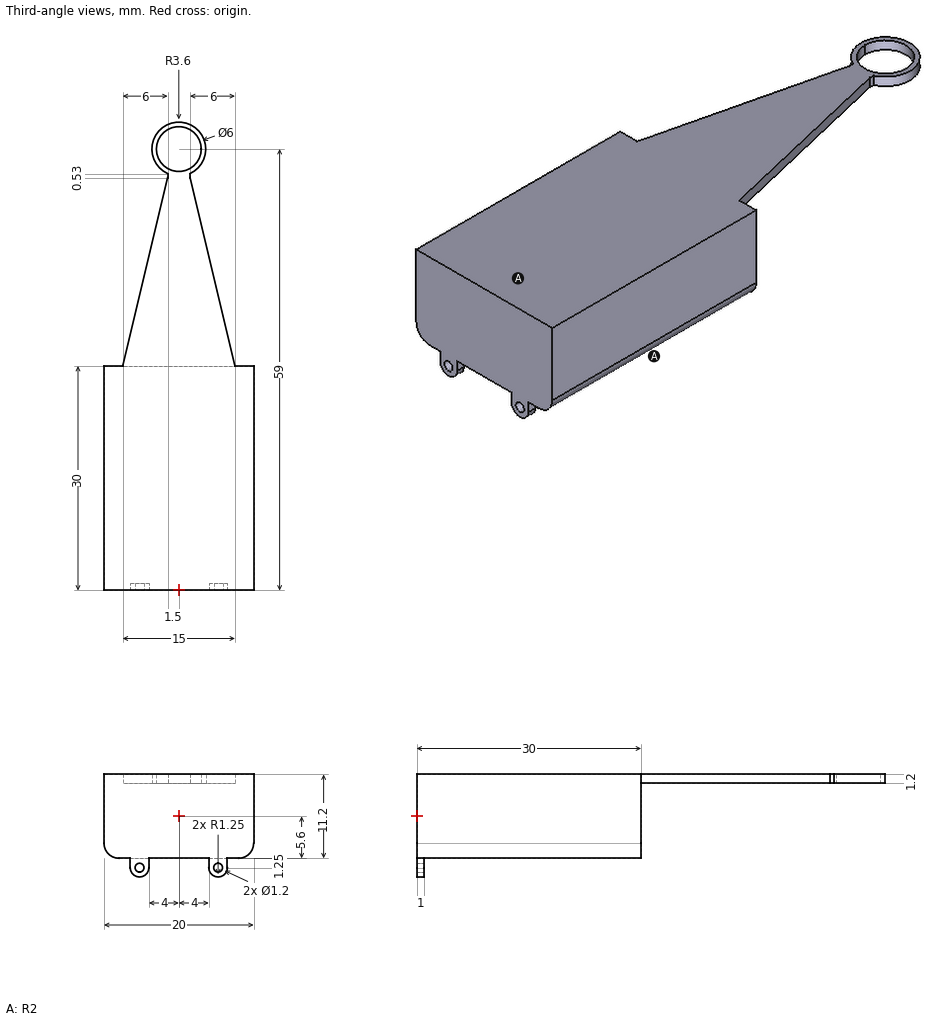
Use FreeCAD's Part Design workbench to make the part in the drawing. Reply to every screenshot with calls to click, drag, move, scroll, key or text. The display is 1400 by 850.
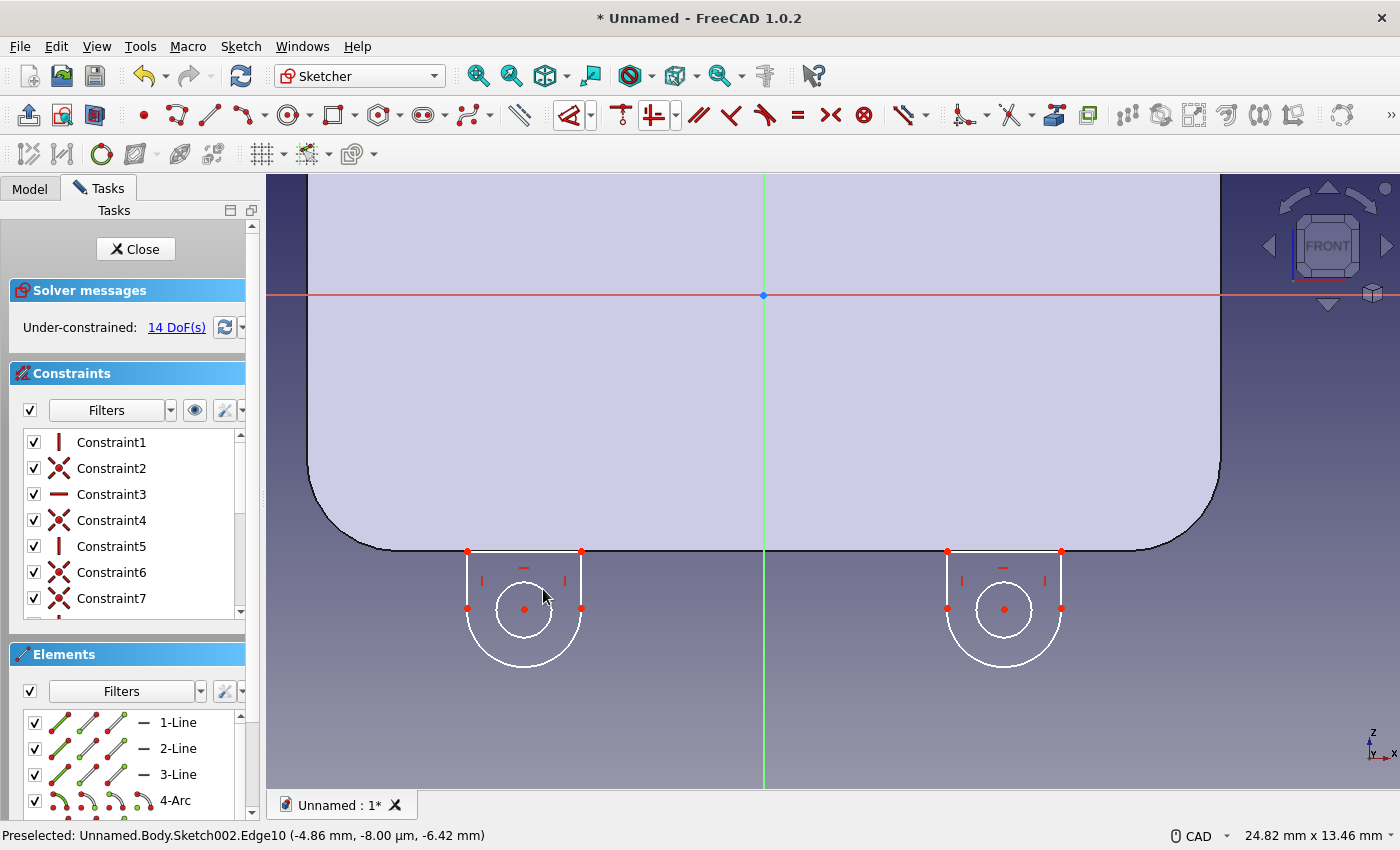
click(1061, 592)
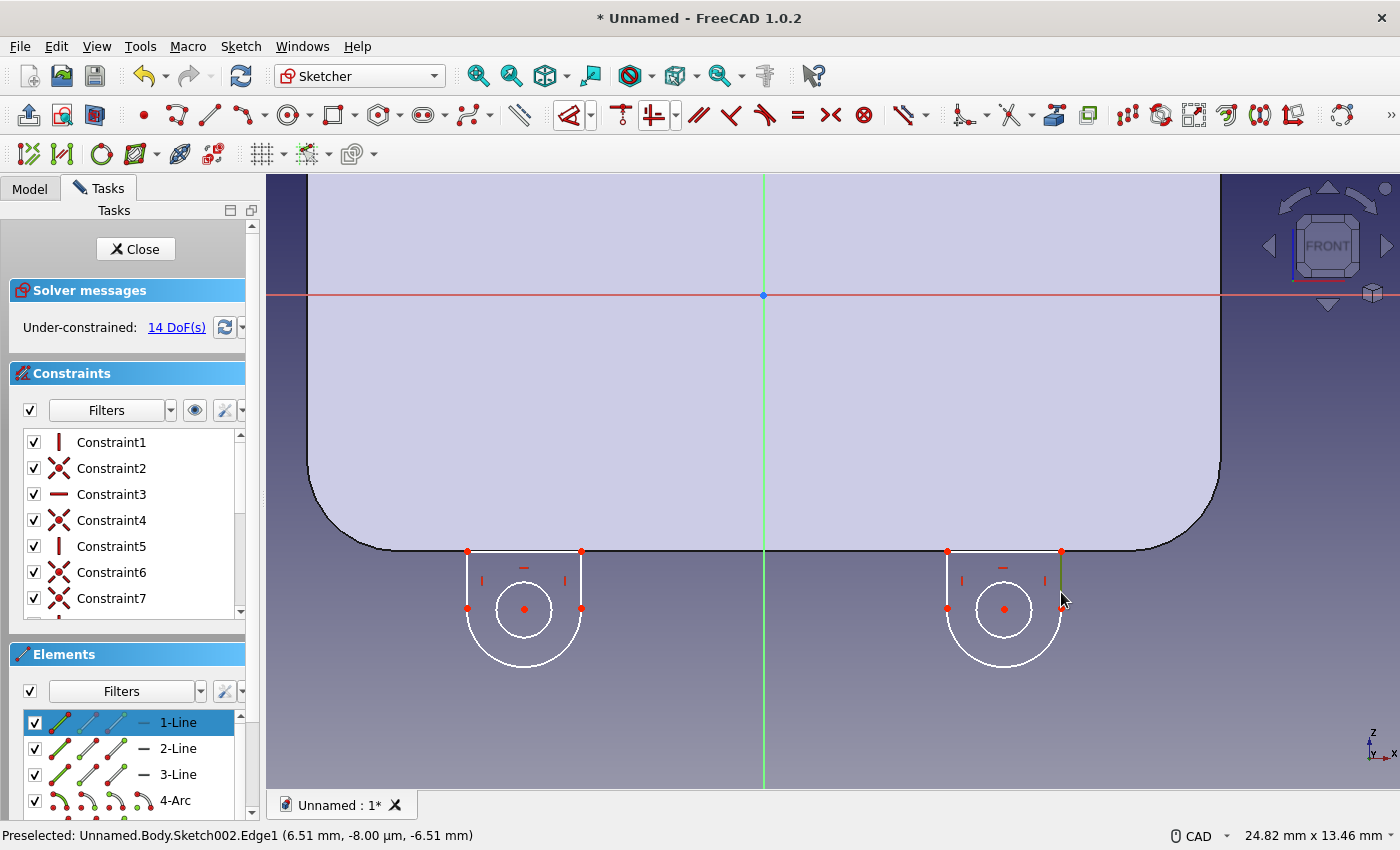
click(970, 656)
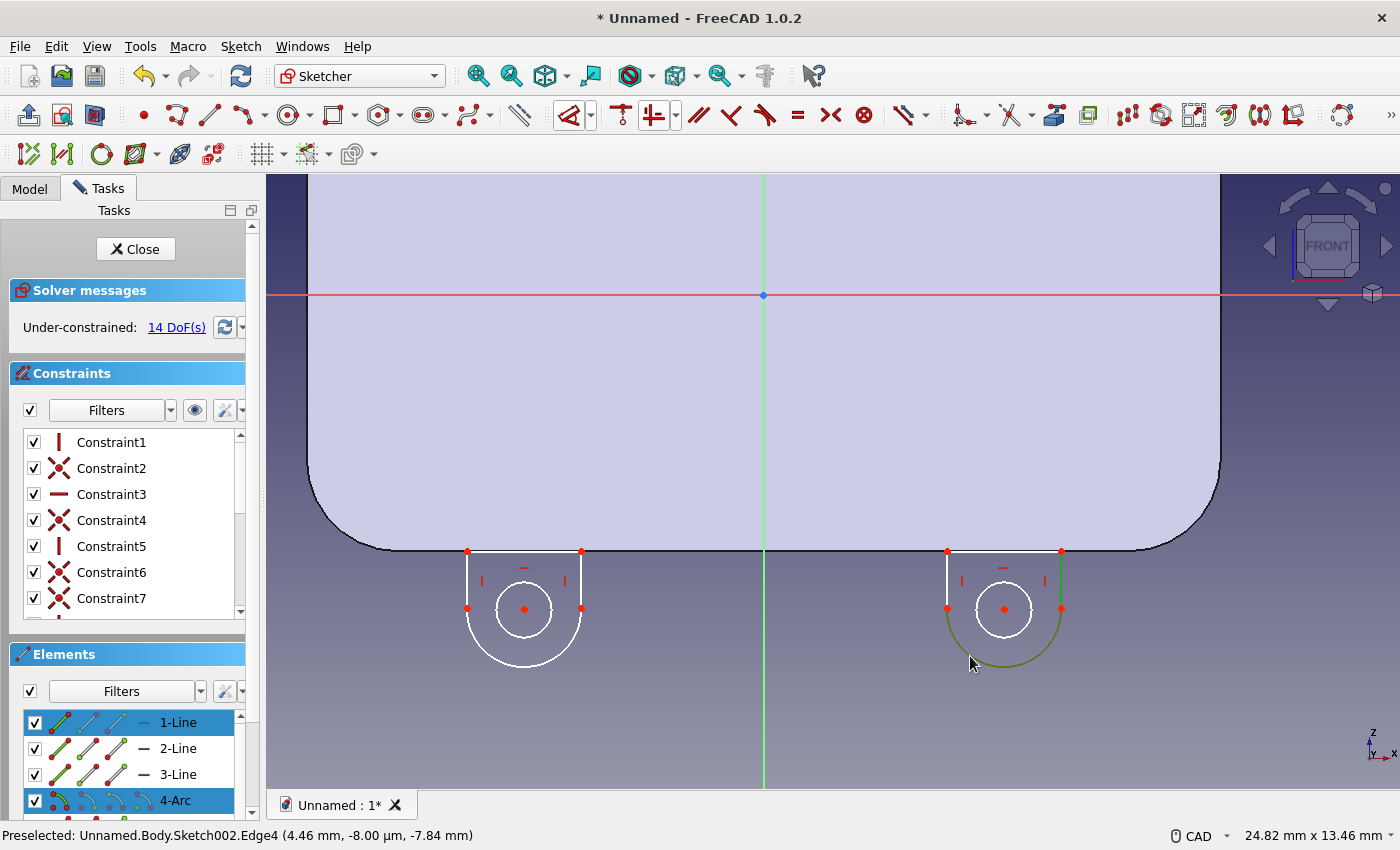
key(t)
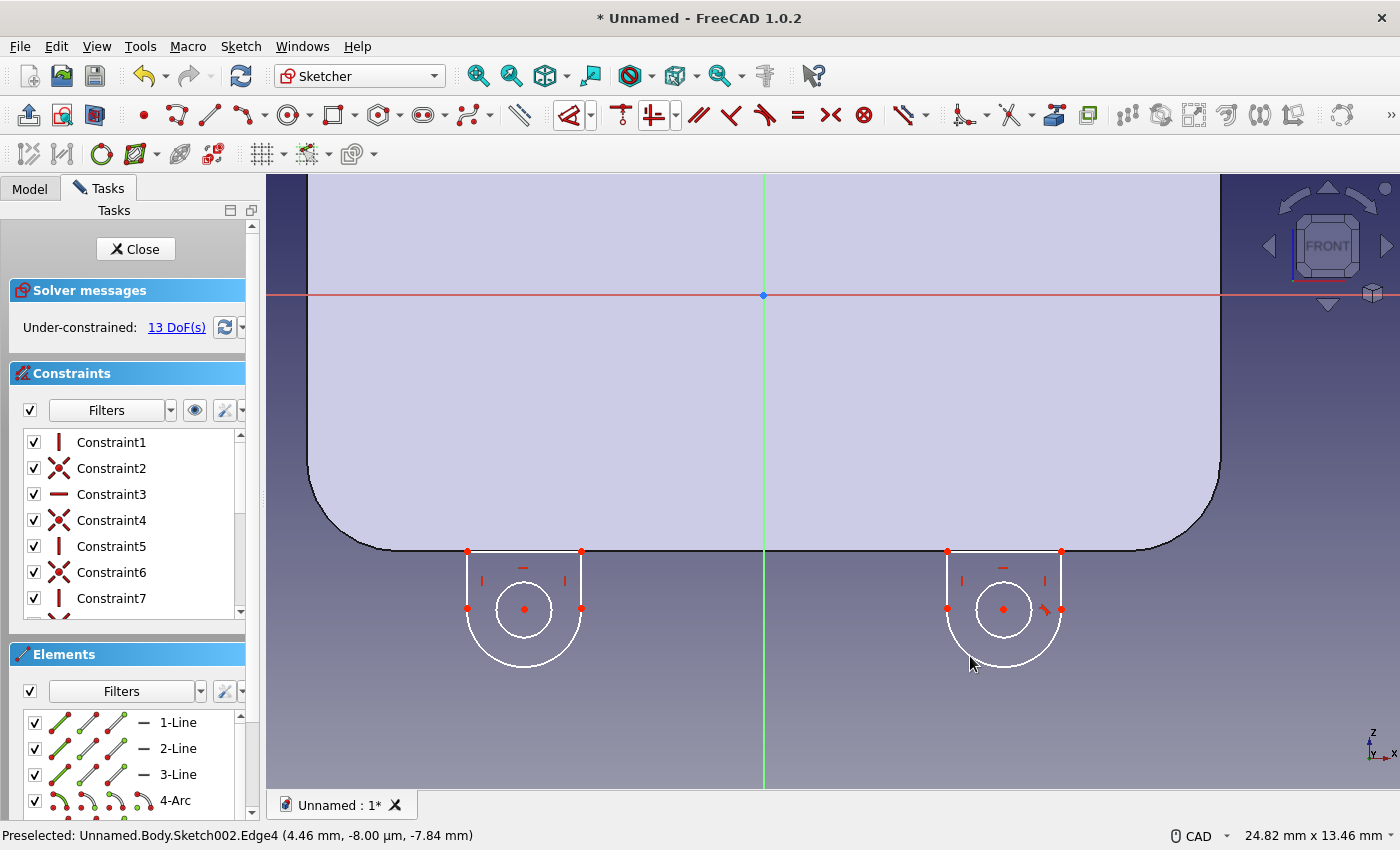
click(947, 569)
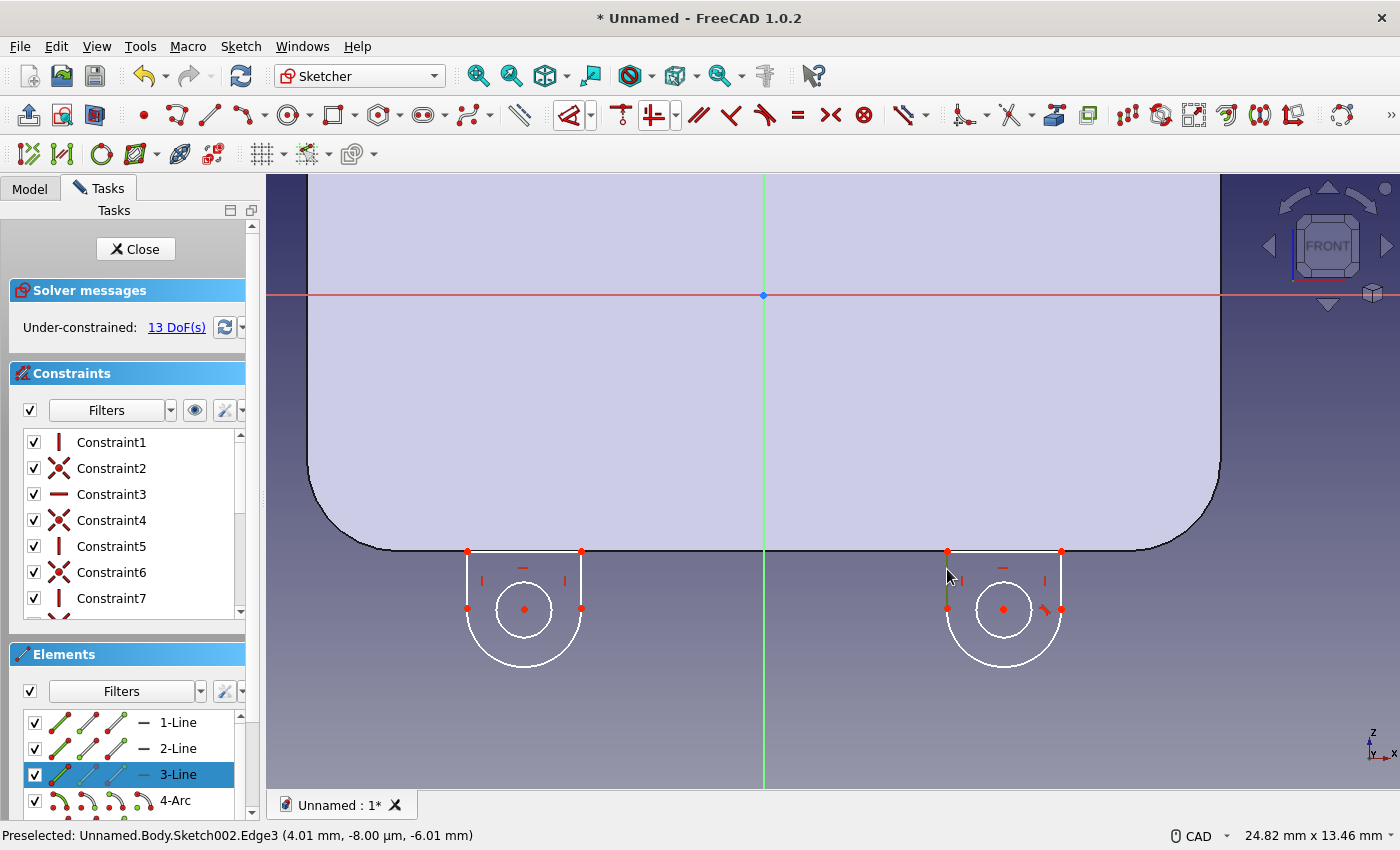
click(970, 656)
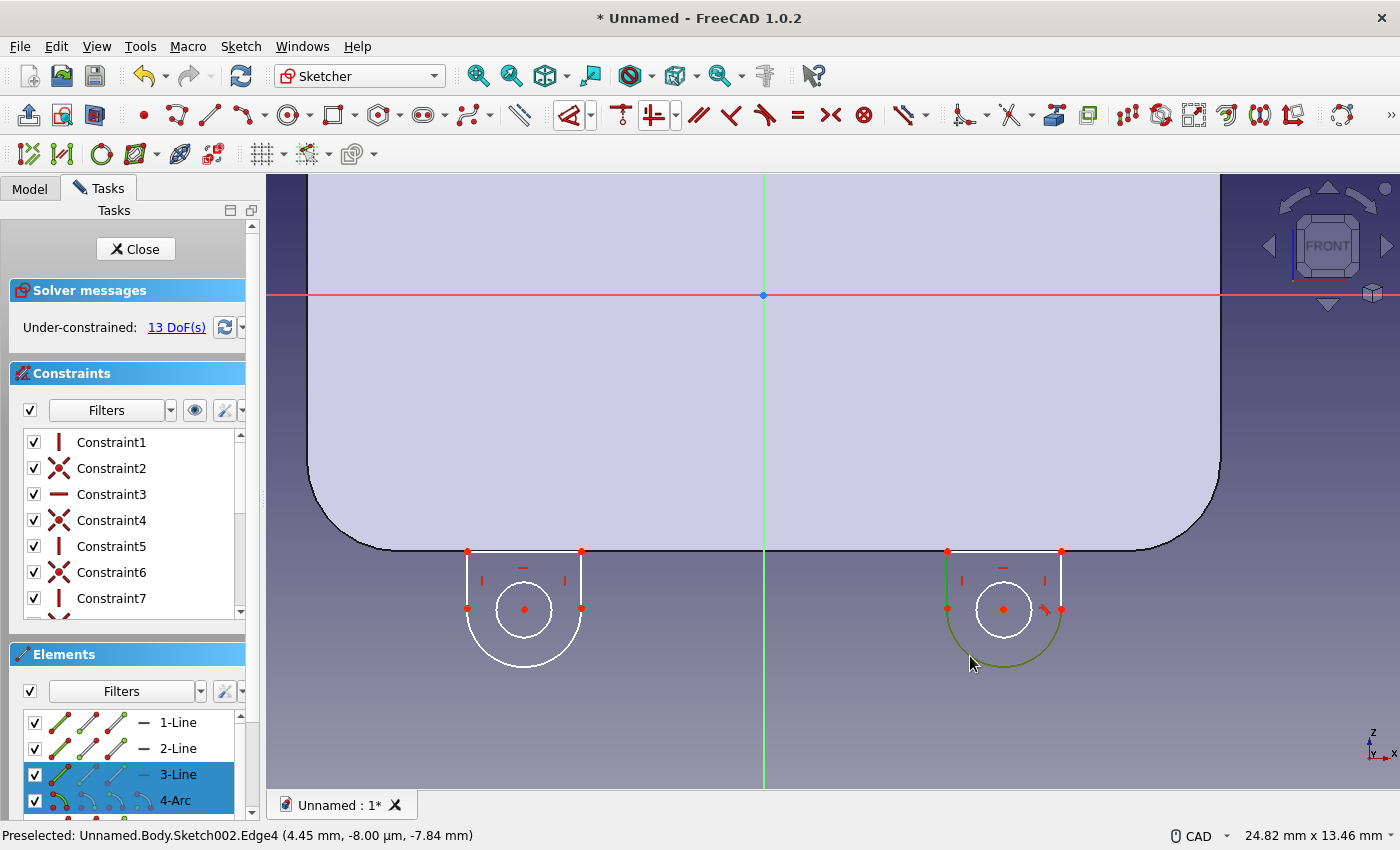
click(765, 116)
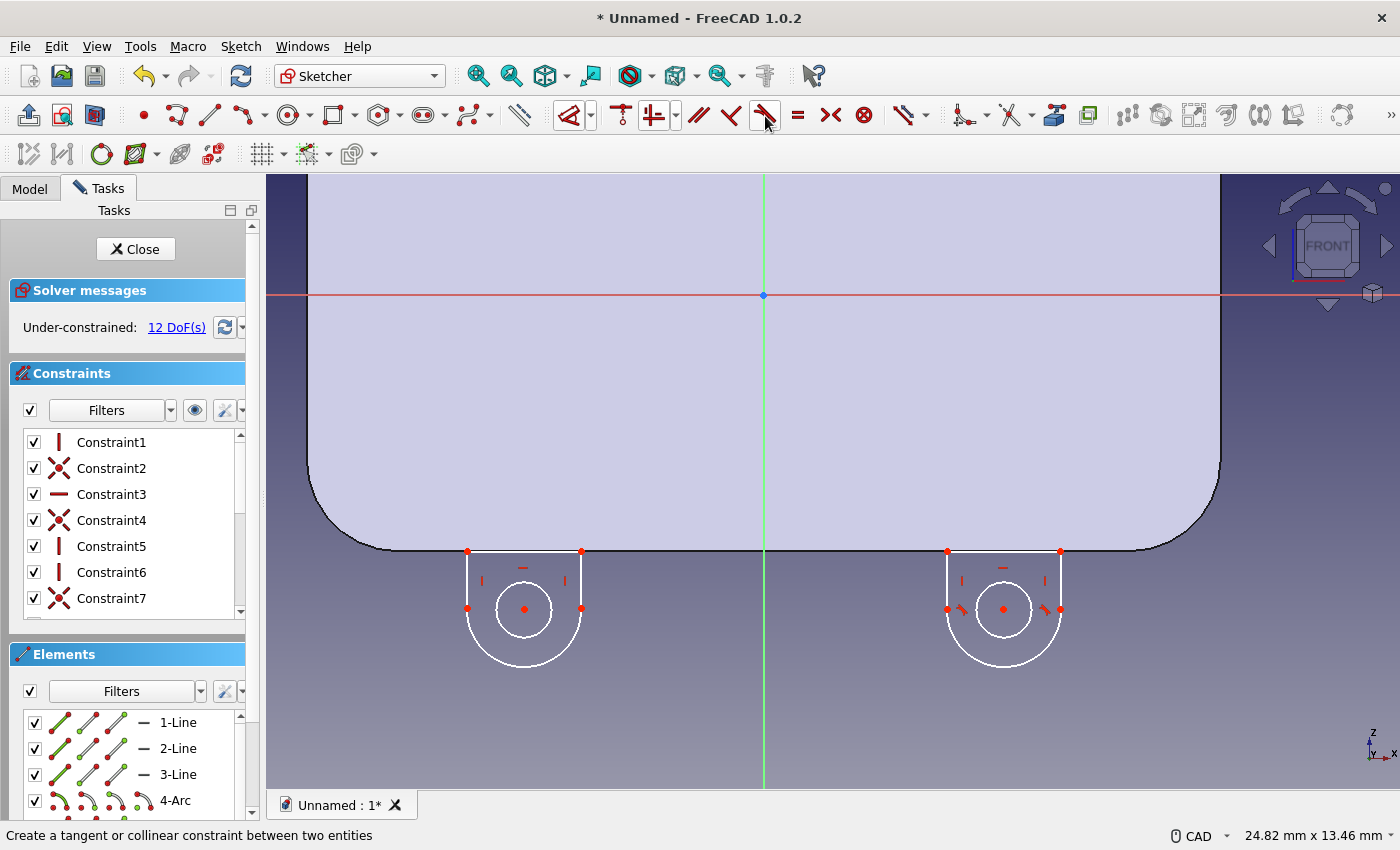
click(581, 592)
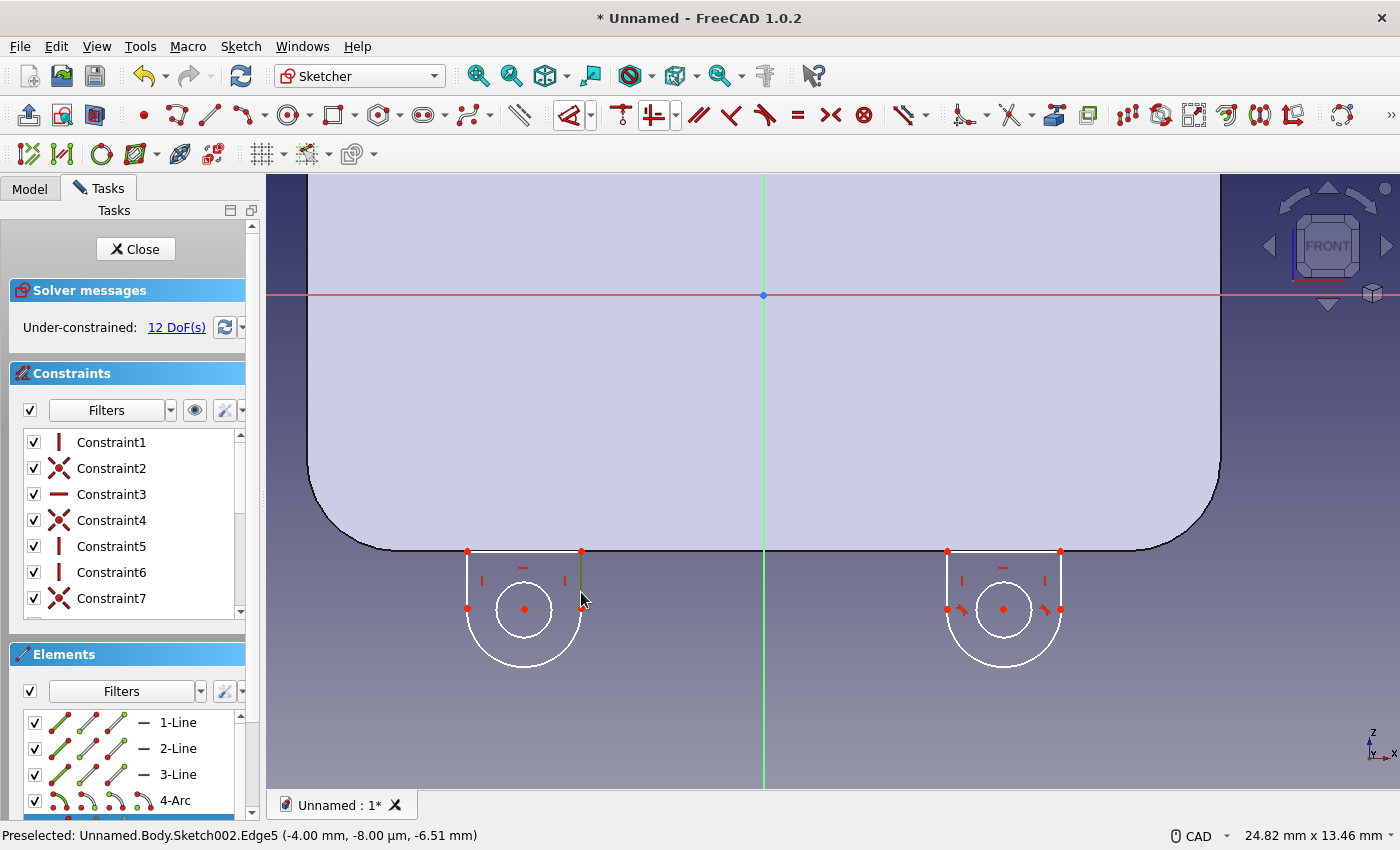
click(490, 656)